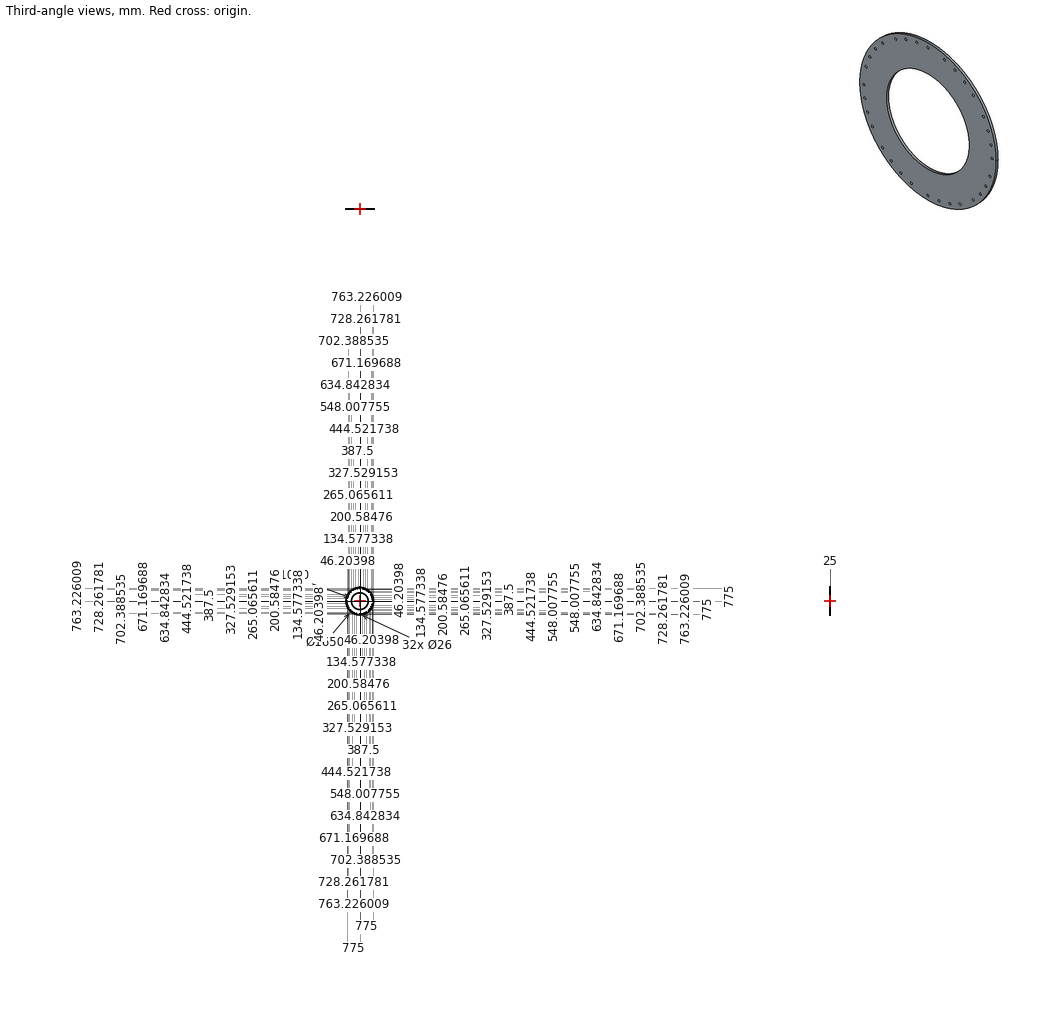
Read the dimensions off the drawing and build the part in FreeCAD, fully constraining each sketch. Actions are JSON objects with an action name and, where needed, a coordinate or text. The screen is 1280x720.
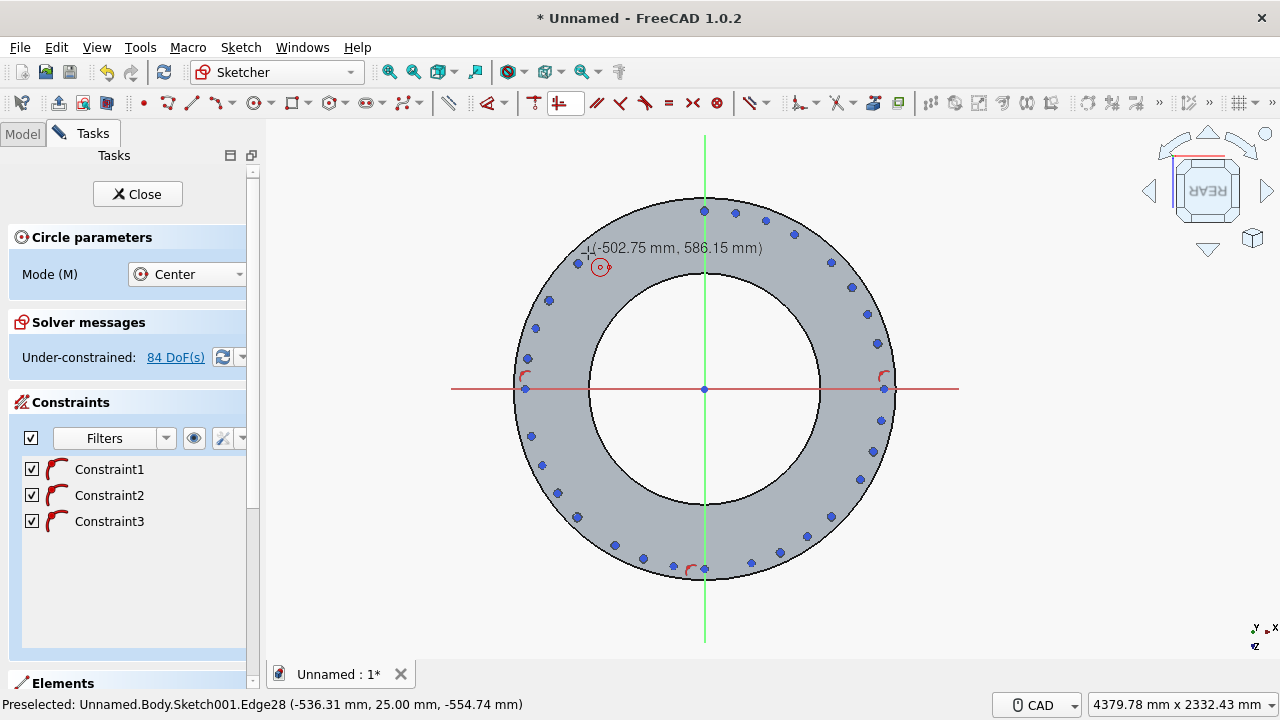
{"action": "left_click", "coordinate": [602, 242]}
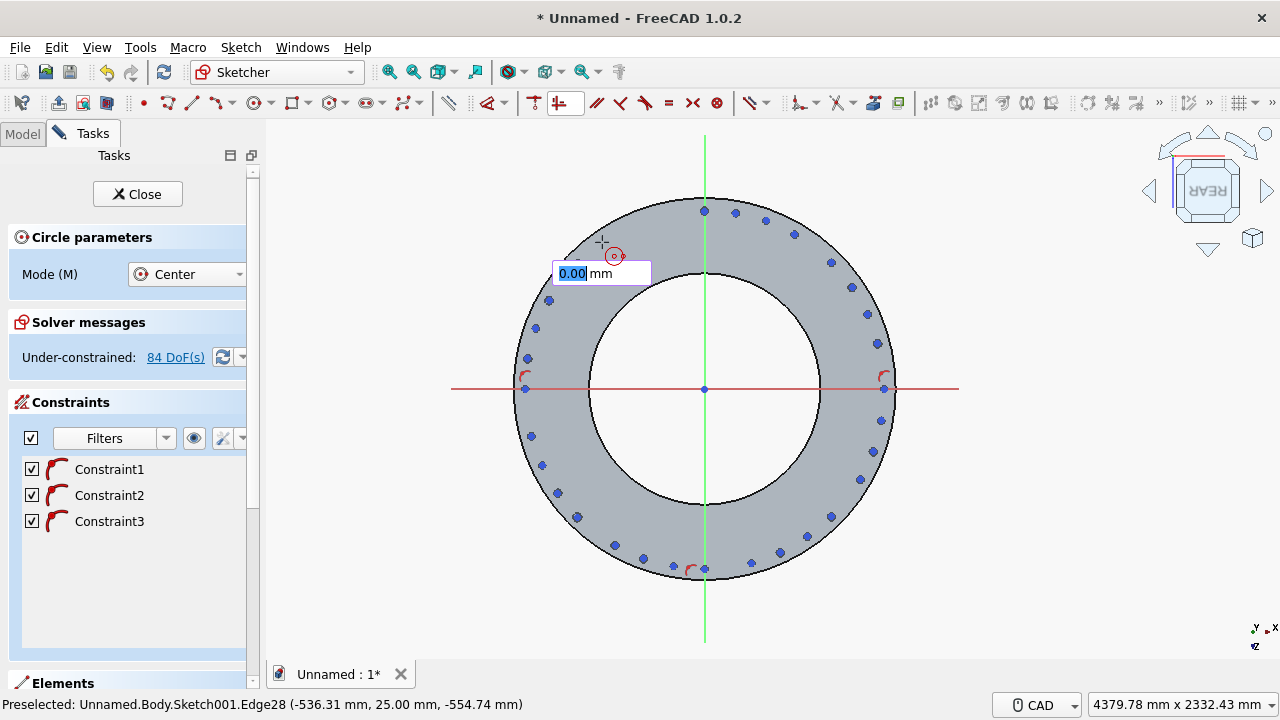
{"action": "scroll", "coordinate": [604, 240], "scroll_direction": "up", "scroll_amount": 9}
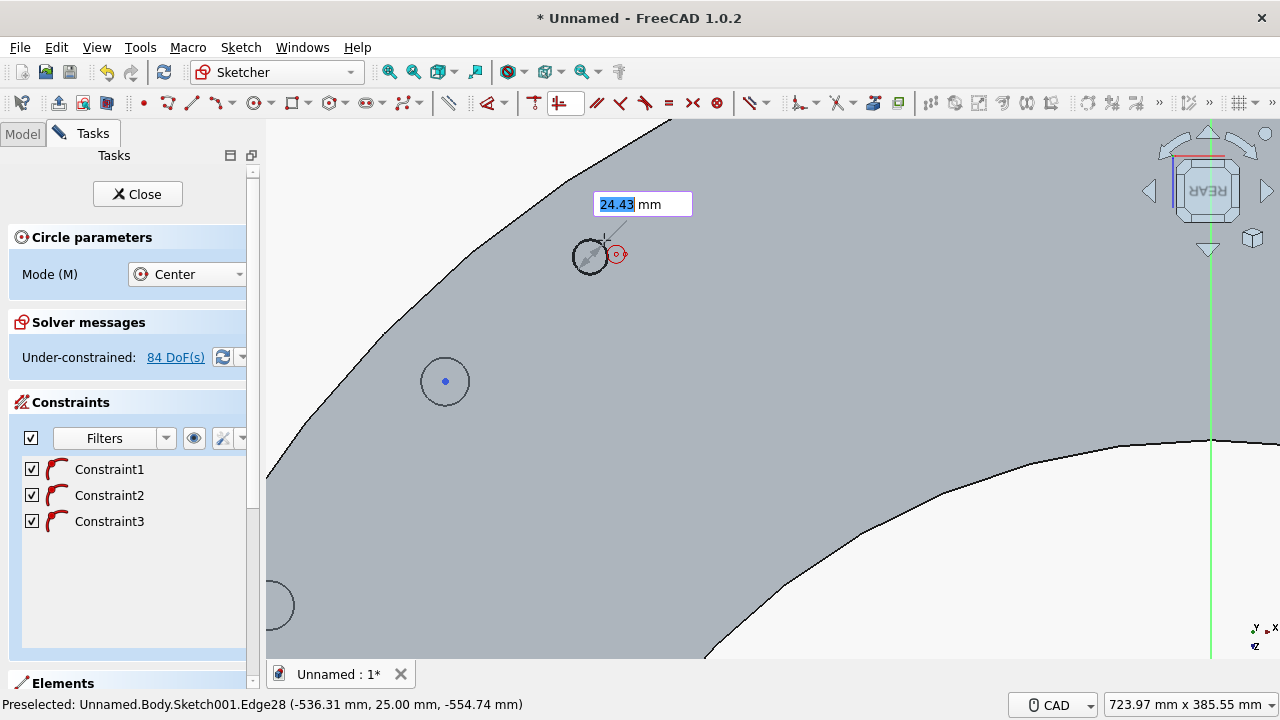
{"action": "left_click", "coordinate": [602, 238]}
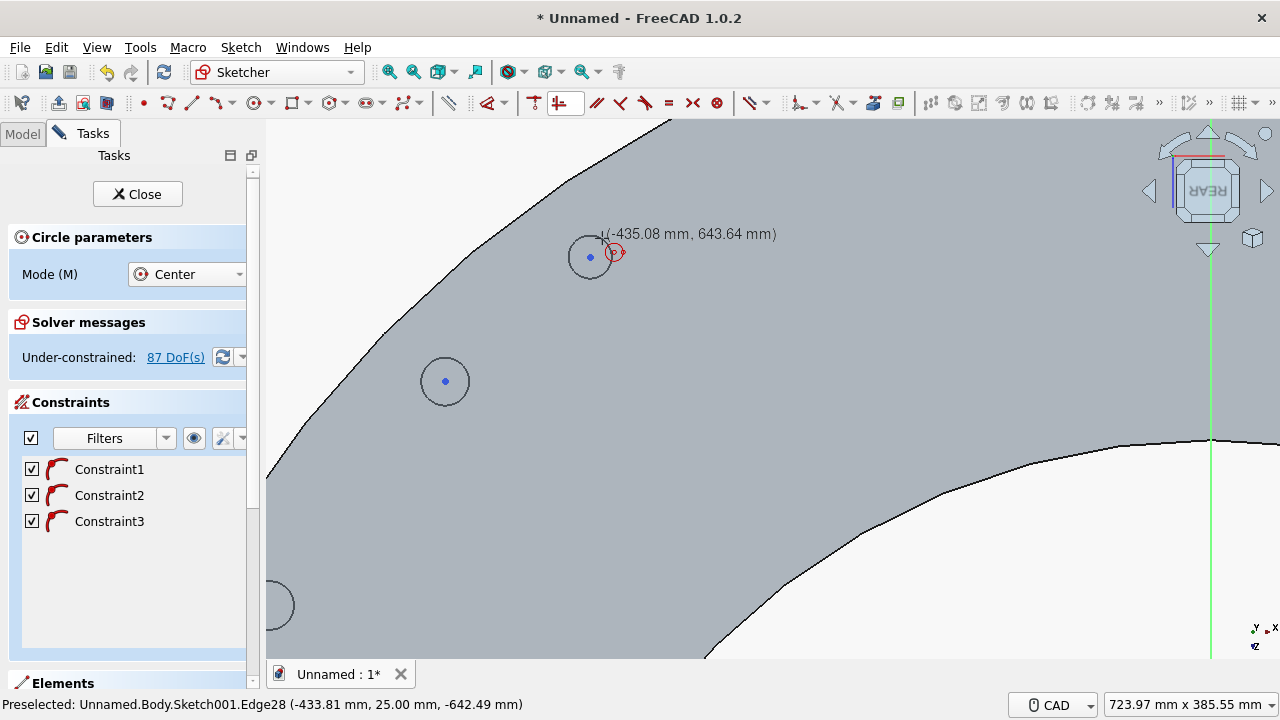
{"action": "scroll", "coordinate": [753, 157], "scroll_direction": "up", "scroll_amount": 2}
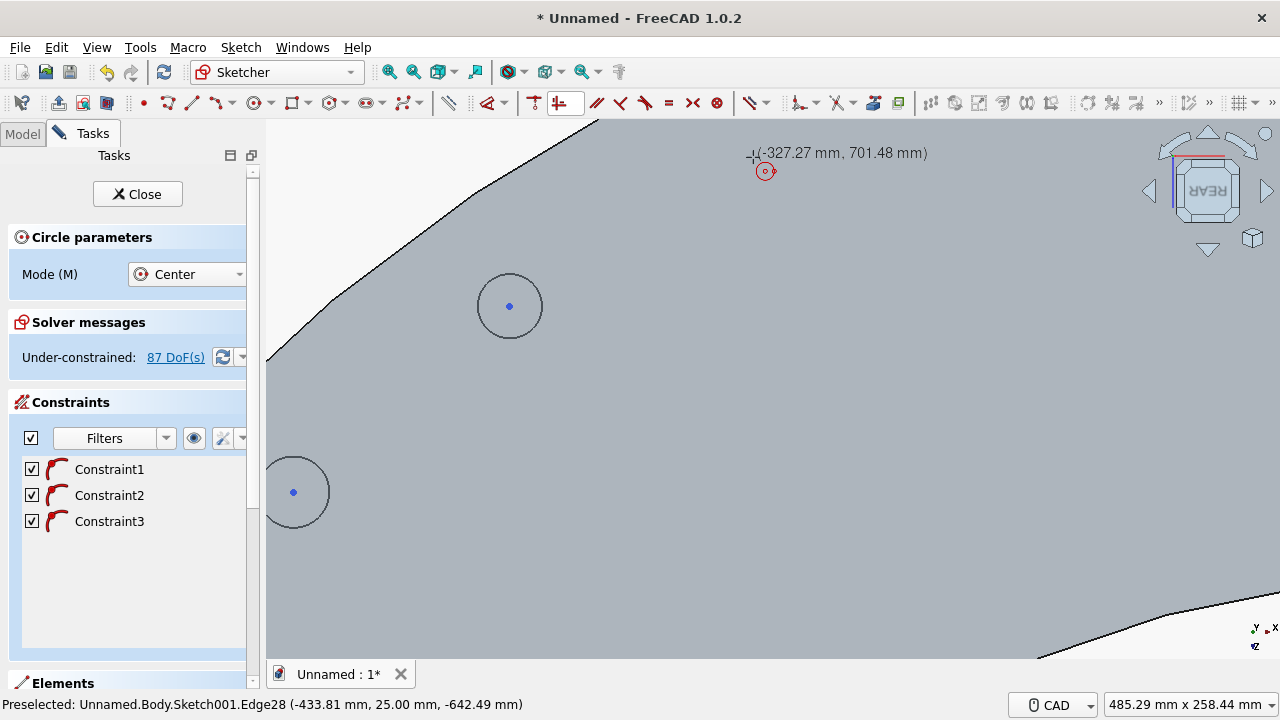
{"action": "scroll", "coordinate": [613, 235], "scroll_direction": "down", "scroll_amount": 11}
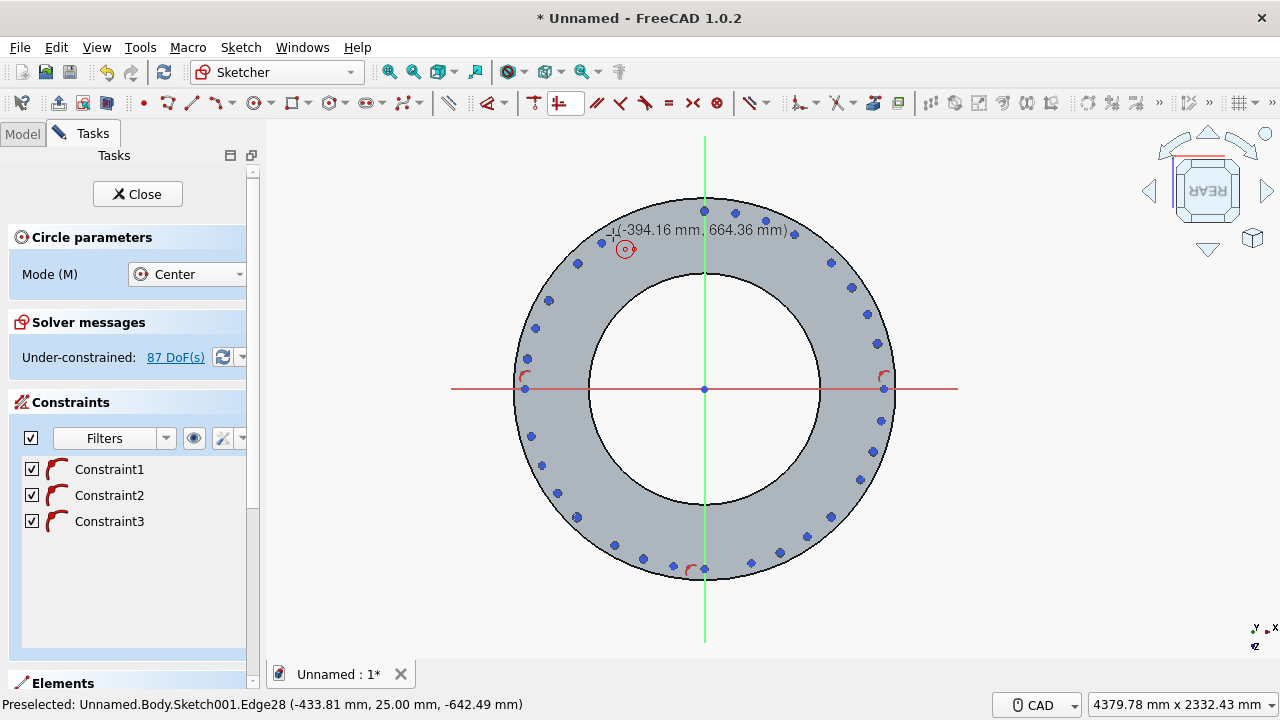
{"action": "left_click", "coordinate": [629, 226]}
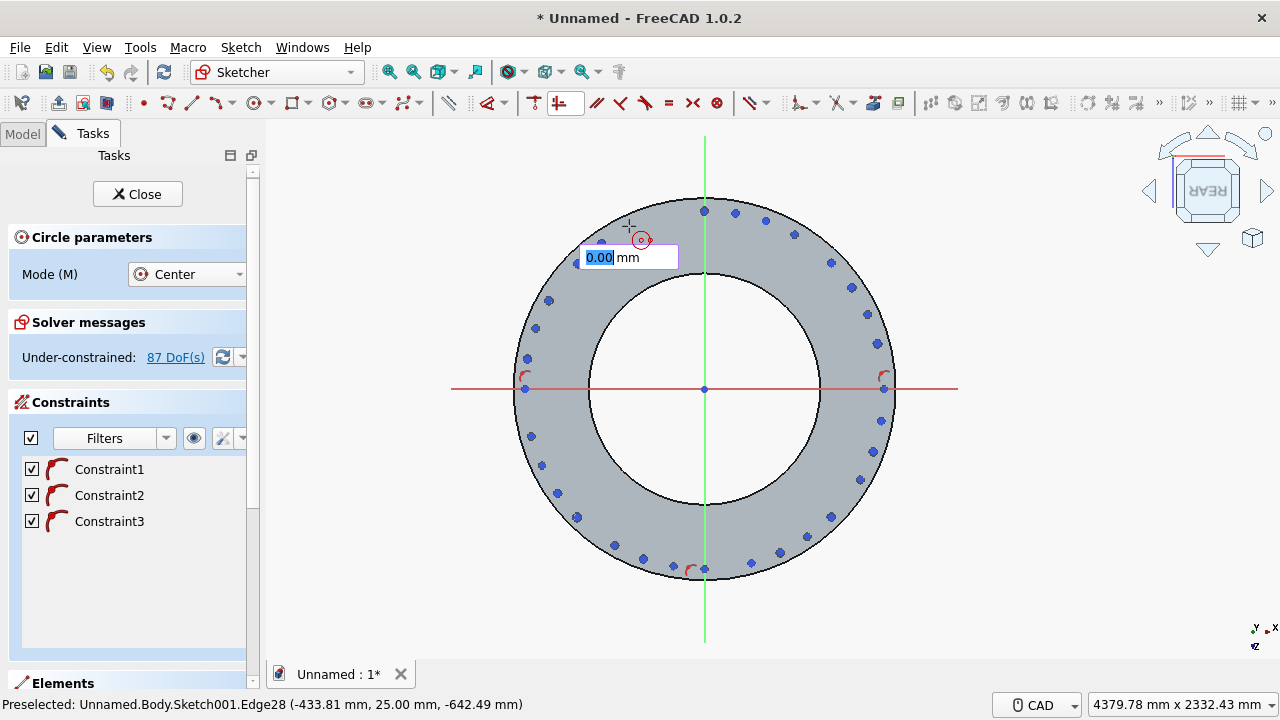
{"action": "scroll", "coordinate": [631, 224], "scroll_direction": "up", "scroll_amount": 9}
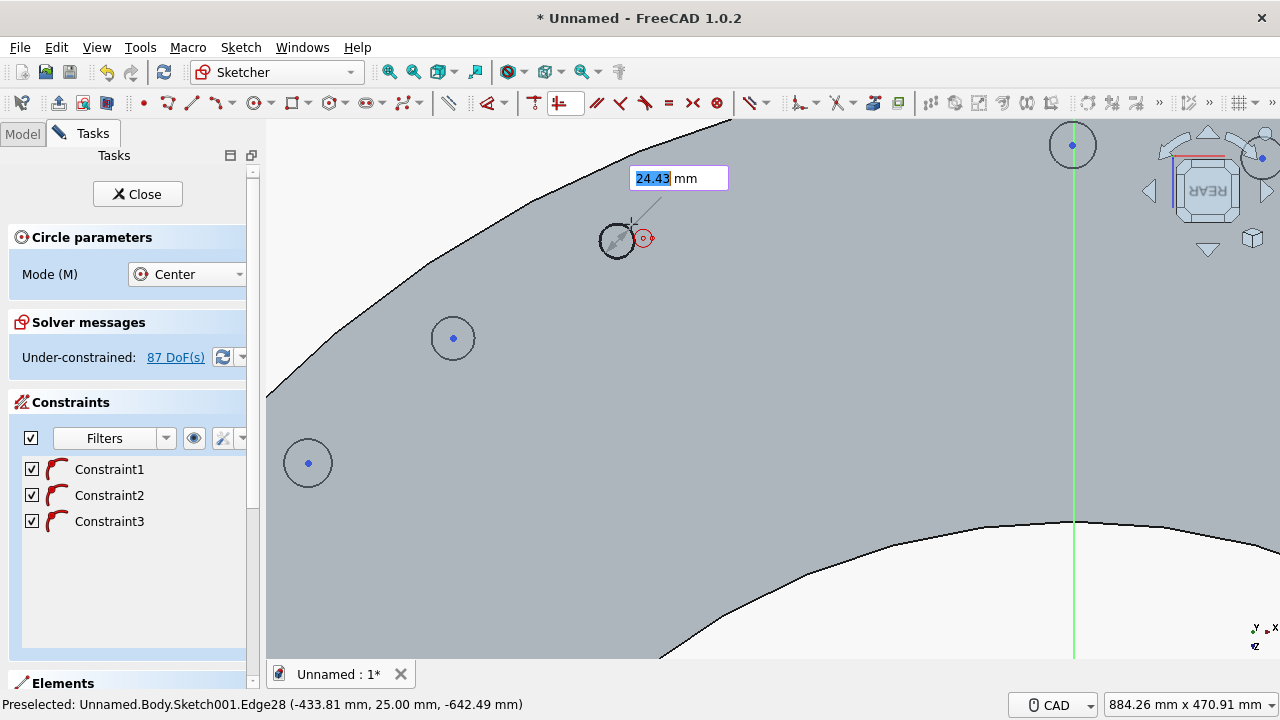
{"action": "left_click", "coordinate": [628, 225]}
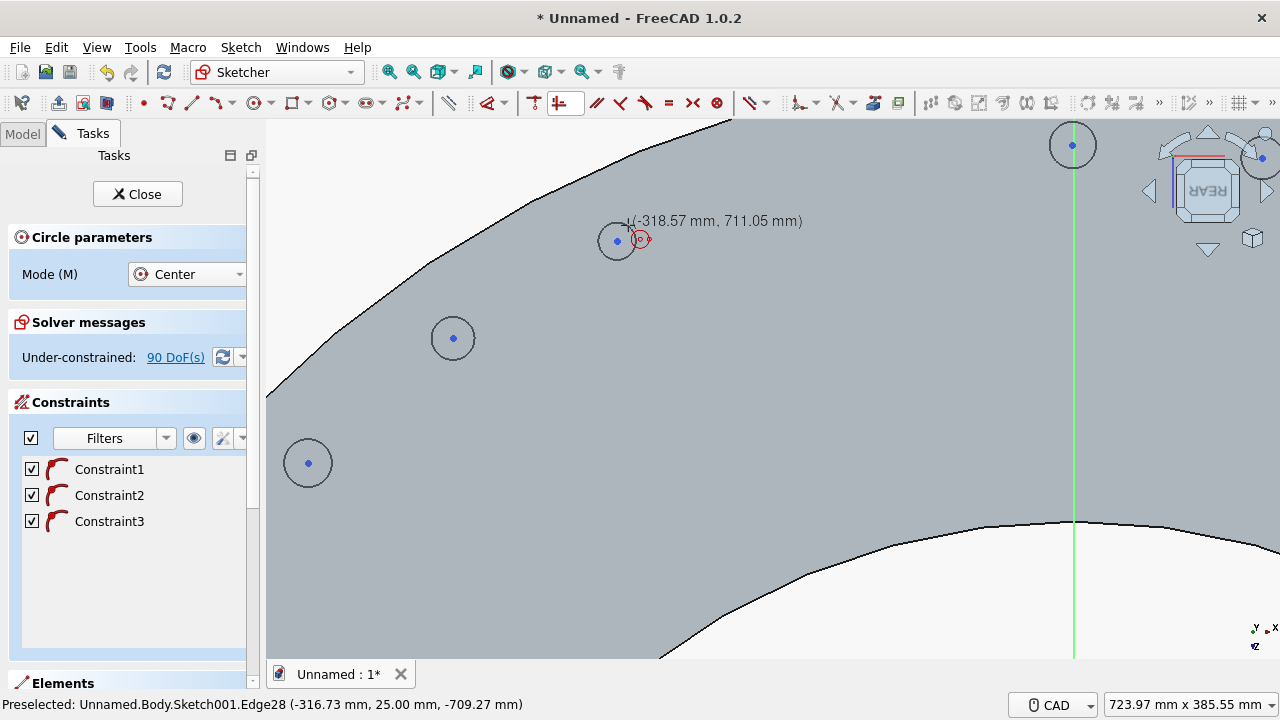
{"action": "scroll", "coordinate": [793, 173], "scroll_direction": "up", "scroll_amount": 2}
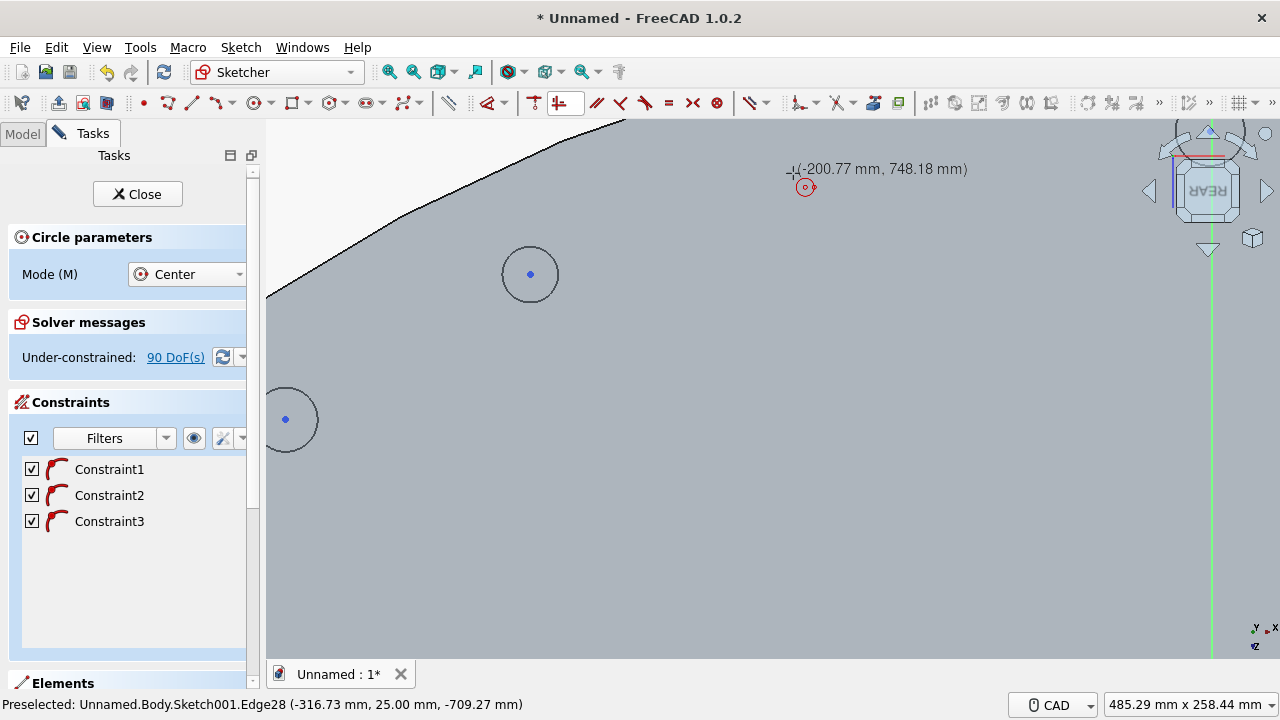
{"action": "scroll", "coordinate": [641, 221], "scroll_direction": "down", "scroll_amount": 11}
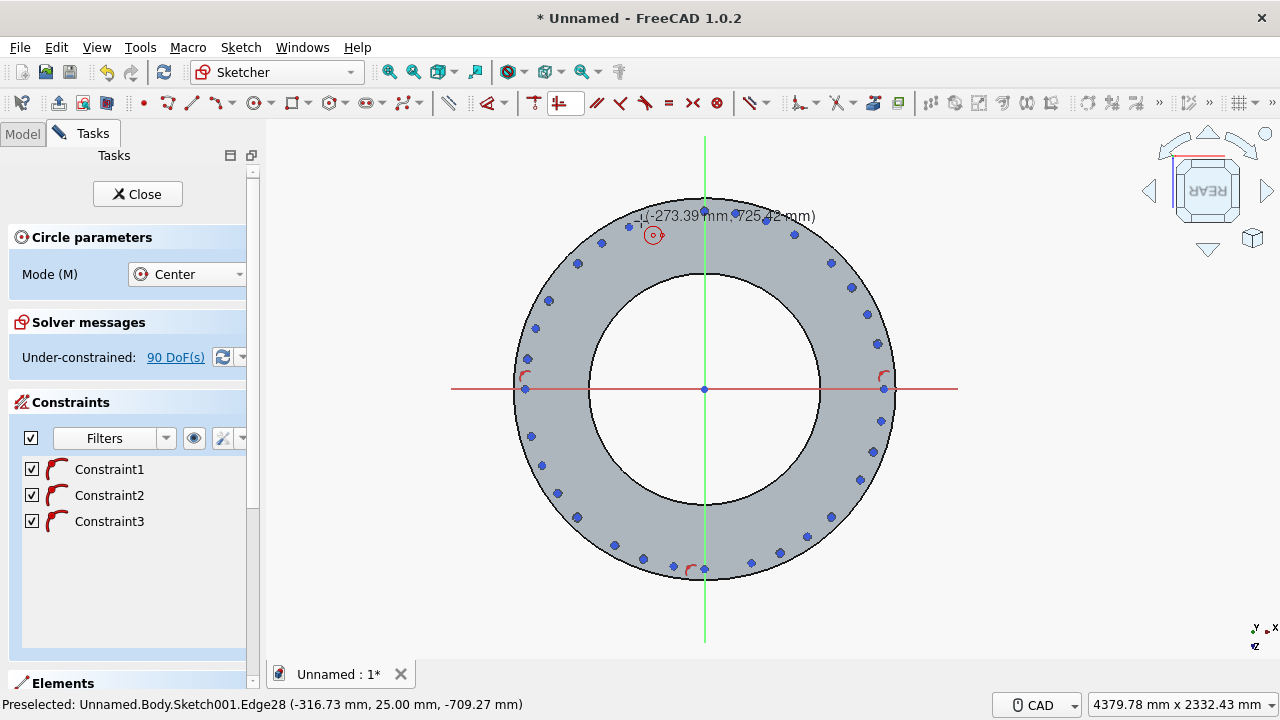
{"action": "left_click", "coordinate": [658, 216]}